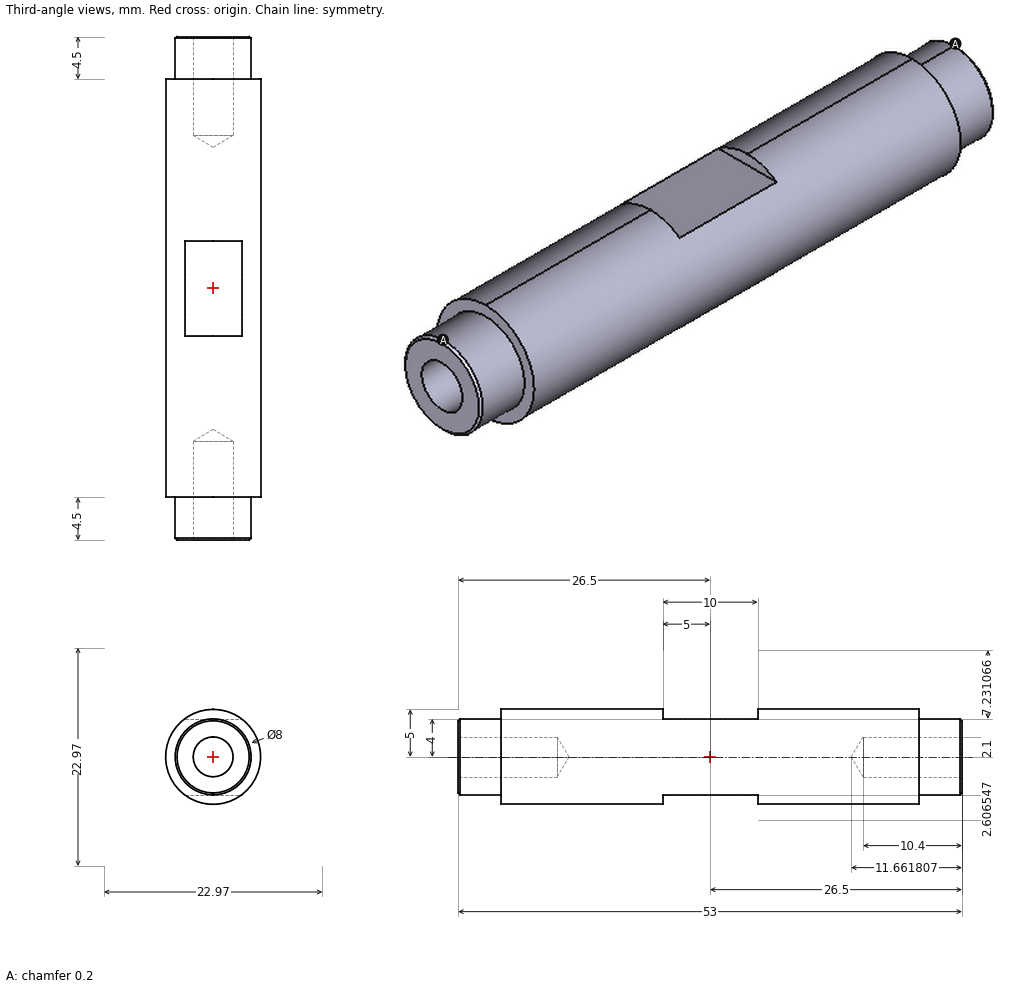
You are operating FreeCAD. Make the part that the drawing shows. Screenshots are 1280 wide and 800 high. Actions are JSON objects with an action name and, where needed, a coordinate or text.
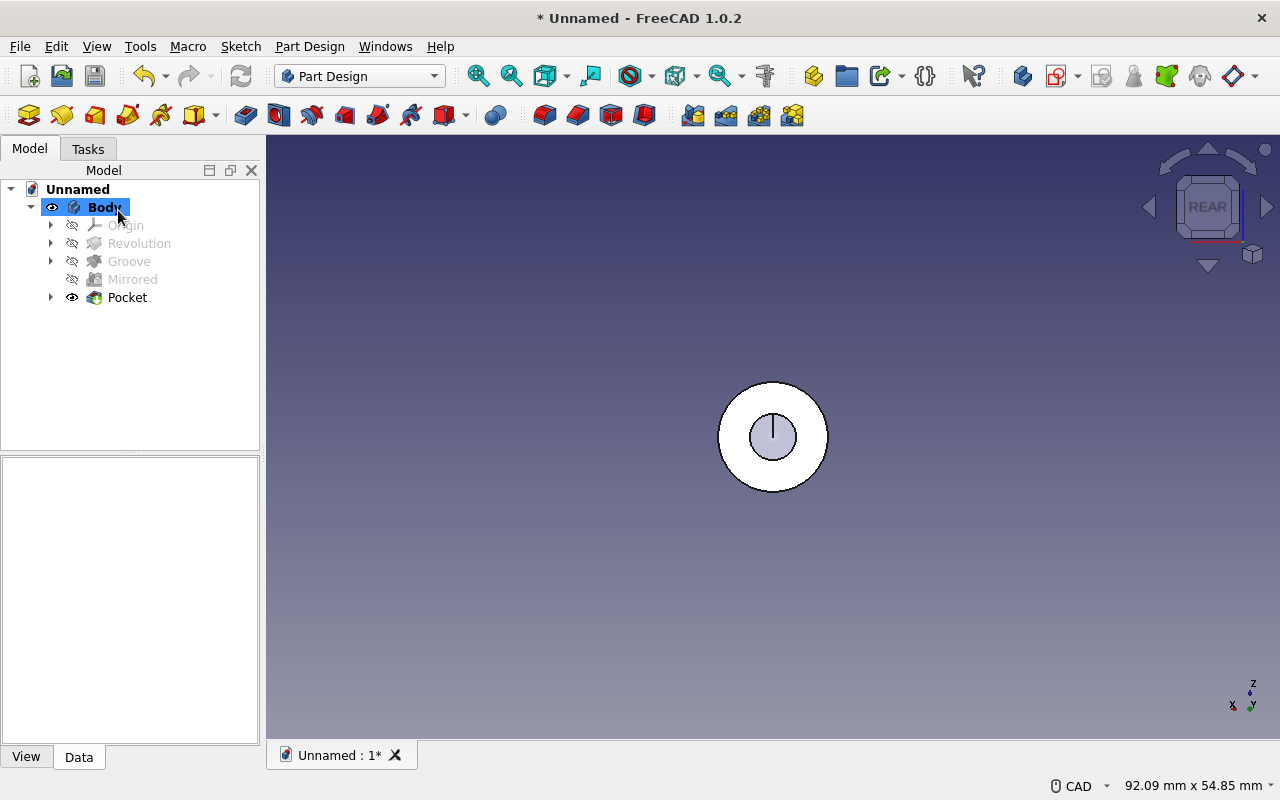
{"action": "left_click", "coordinate": [479, 76]}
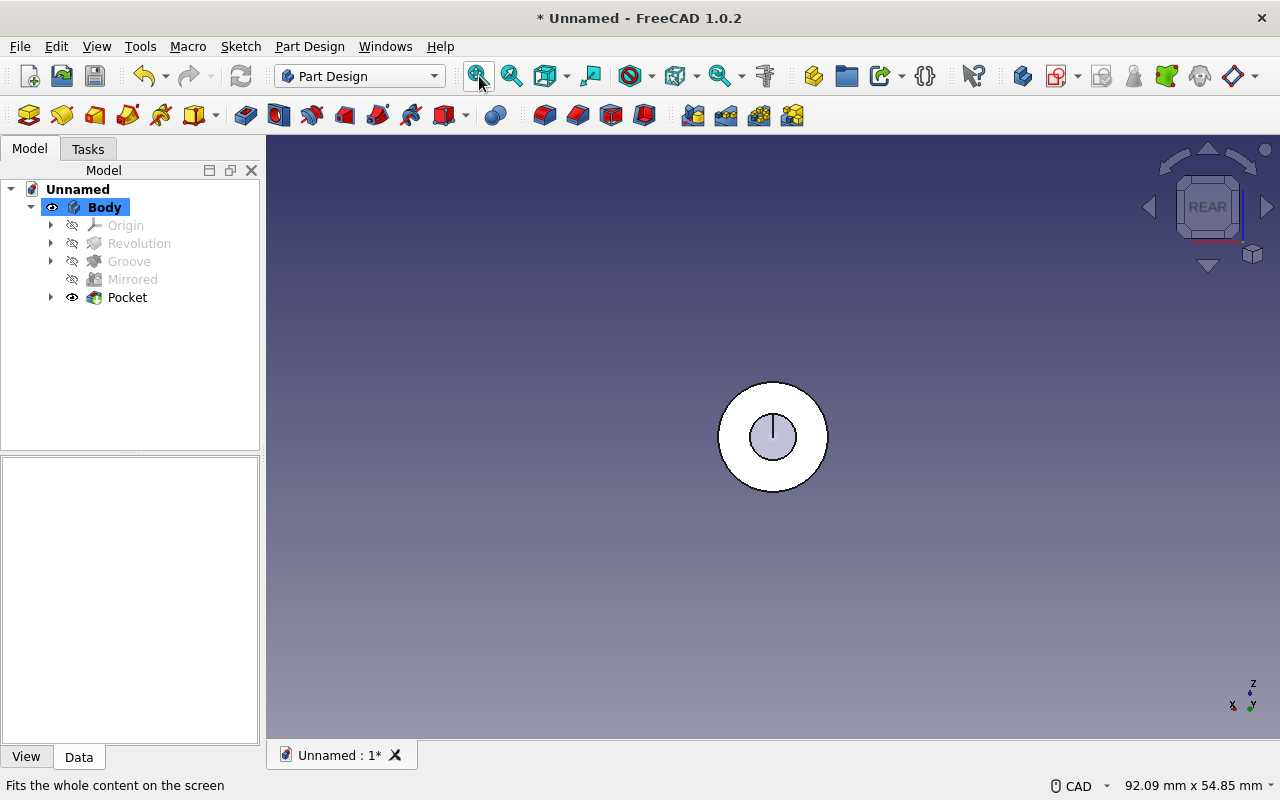
{"action": "left_click", "coordinate": [757, 467]}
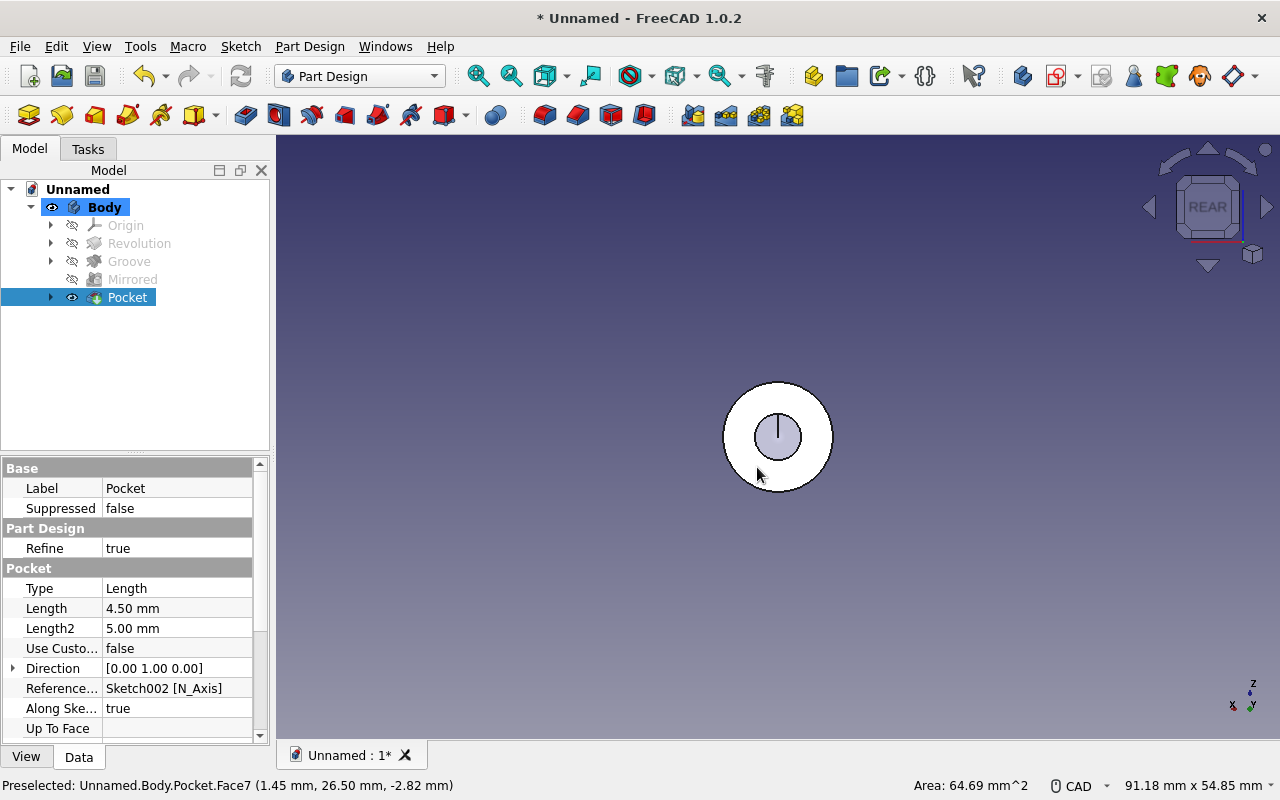
{"action": "left_click", "coordinate": [1056, 76]}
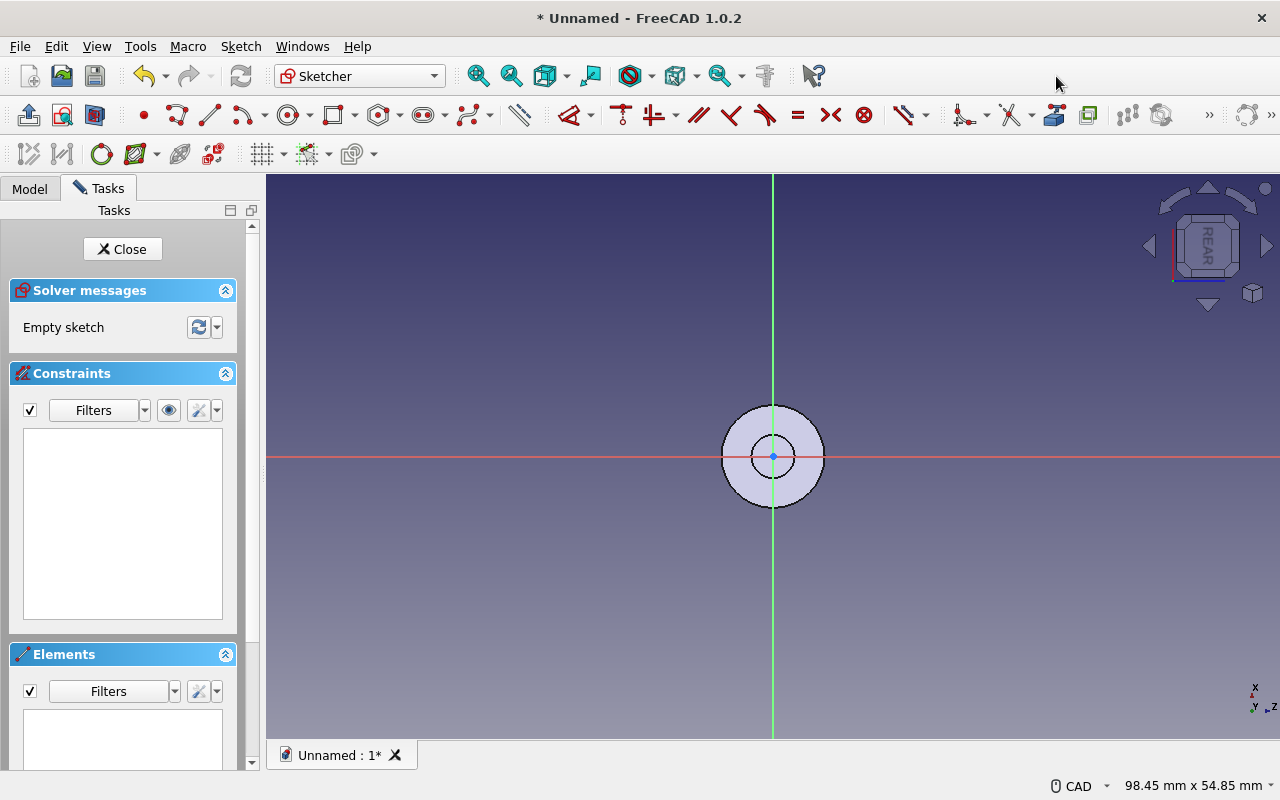
{"action": "scroll", "coordinate": [912, 456], "scroll_direction": "up", "scroll_amount": 2}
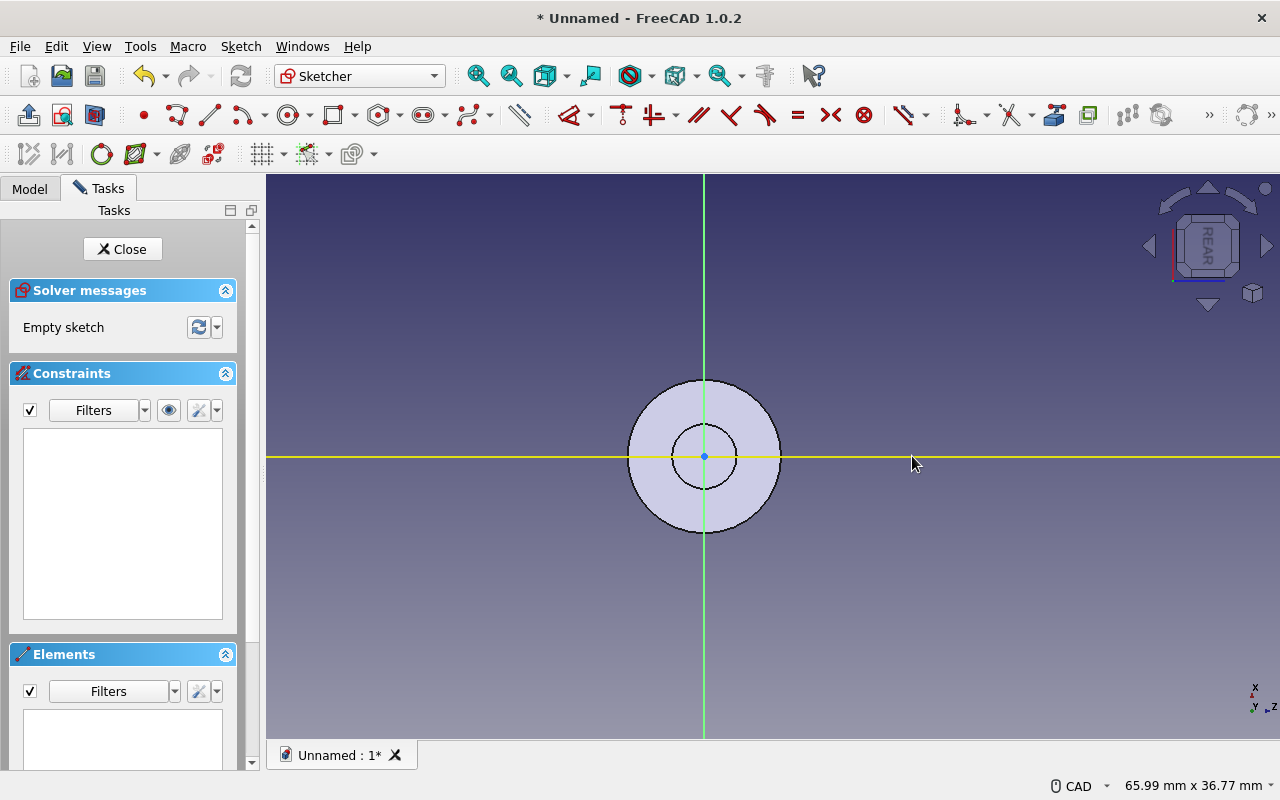
{"action": "left_click", "coordinate": [354, 116]}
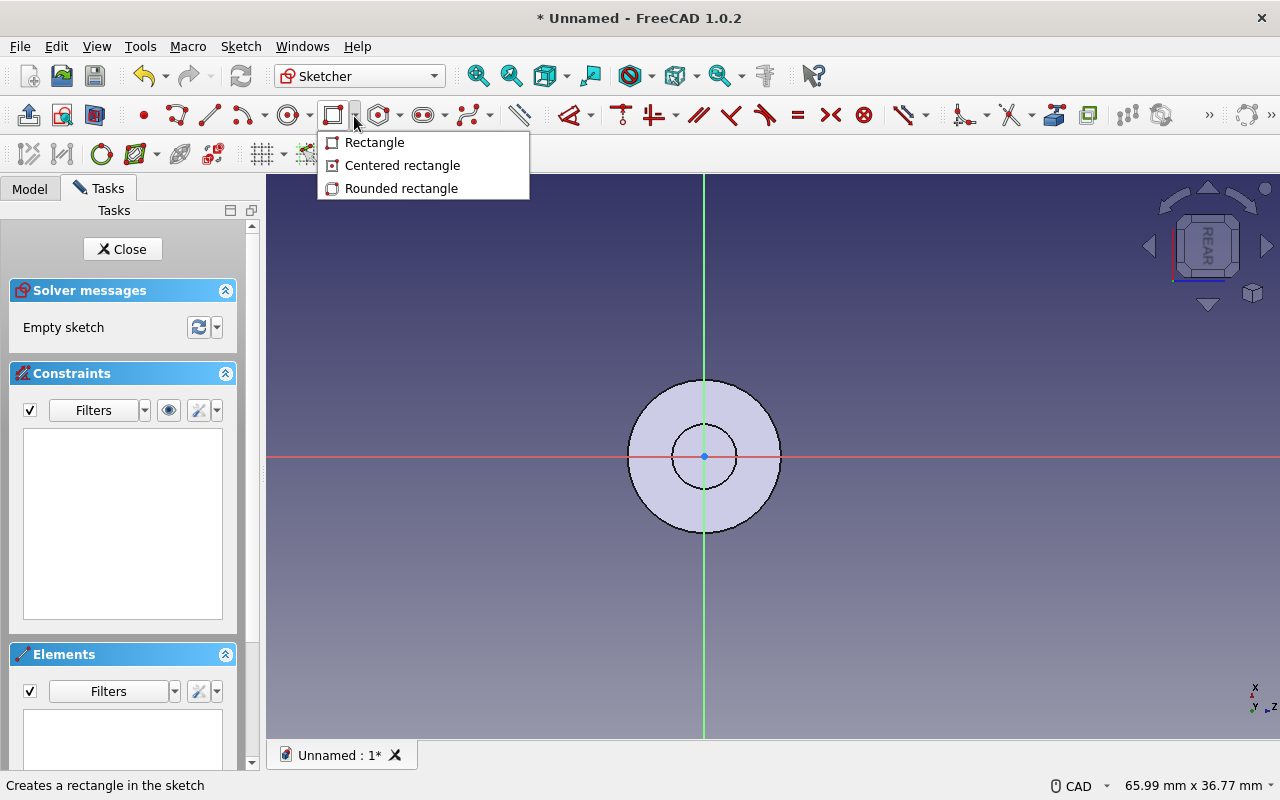
{"action": "left_click", "coordinate": [424, 166]}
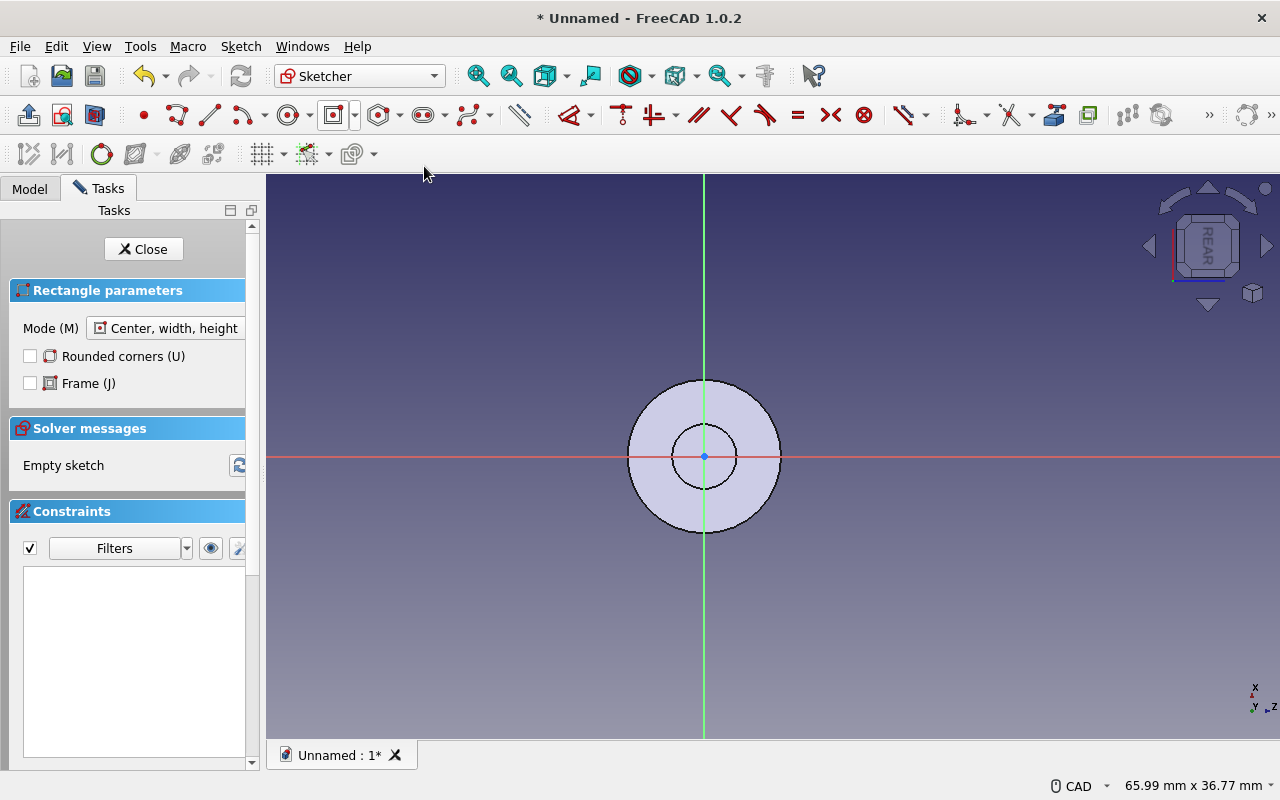
{"action": "left_click", "coordinate": [704, 456]}
{"action": "mouse_move", "coordinate": [881, 280]}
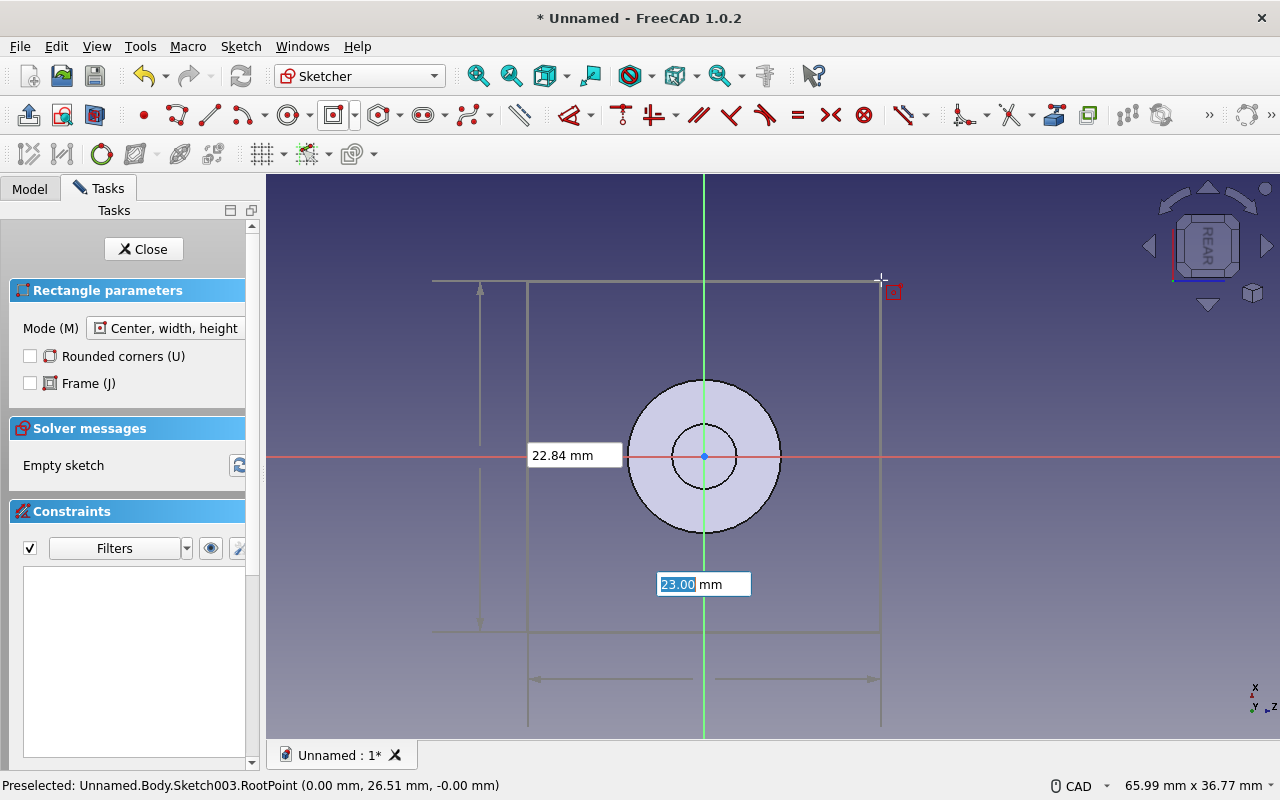
{"action": "type", "text": "22.97"}
{"action": "key", "text": "Tab"}
{"action": "type", "text": "22.97"}
{"action": "key", "text": "Return"}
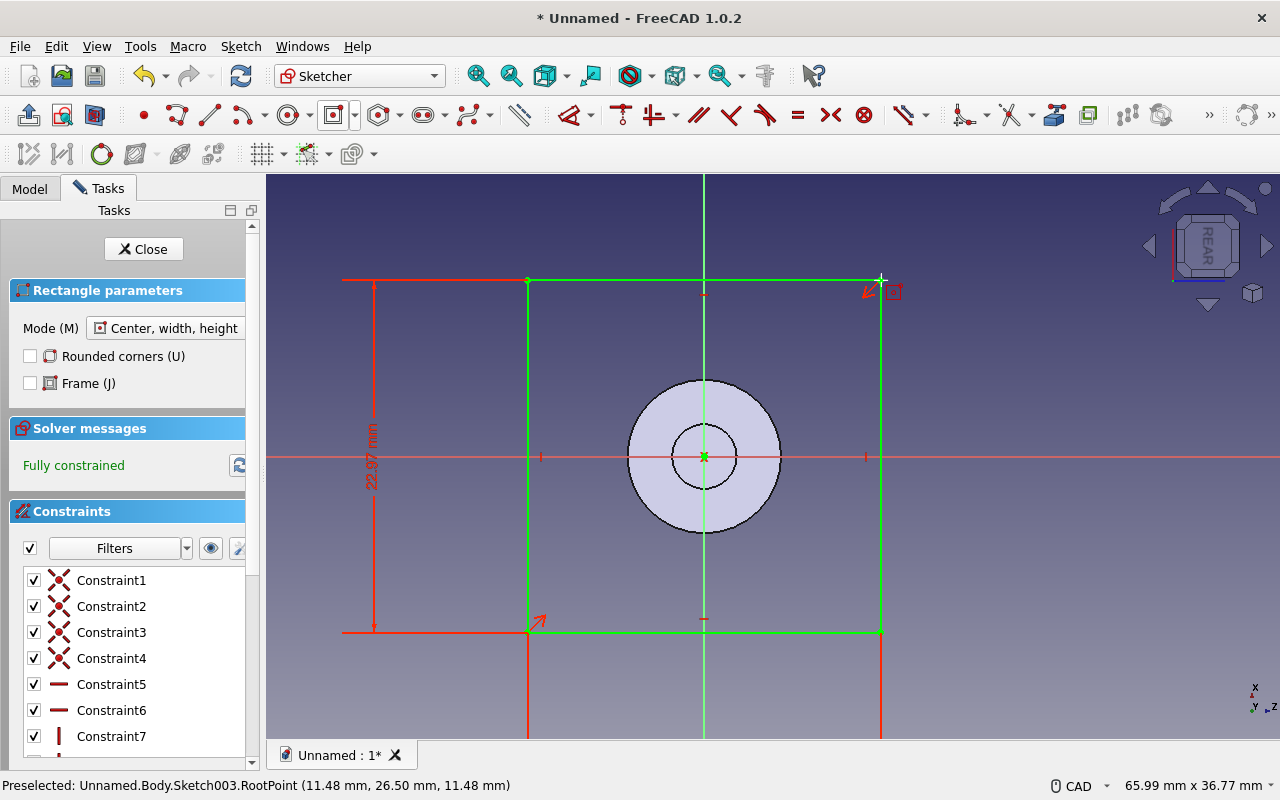
{"action": "left_click", "coordinate": [288, 116]}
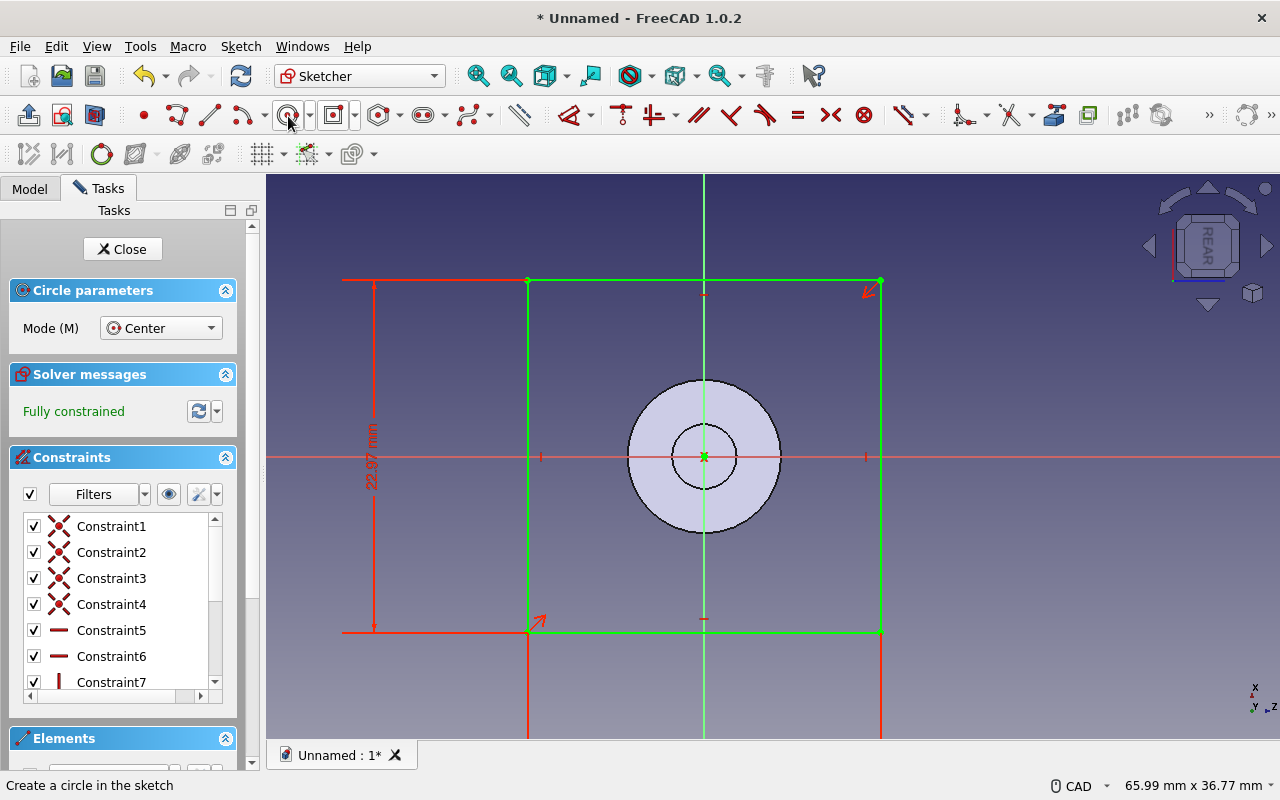
{"action": "left_click", "coordinate": [704, 456]}
{"action": "mouse_move", "coordinate": [748, 413]}